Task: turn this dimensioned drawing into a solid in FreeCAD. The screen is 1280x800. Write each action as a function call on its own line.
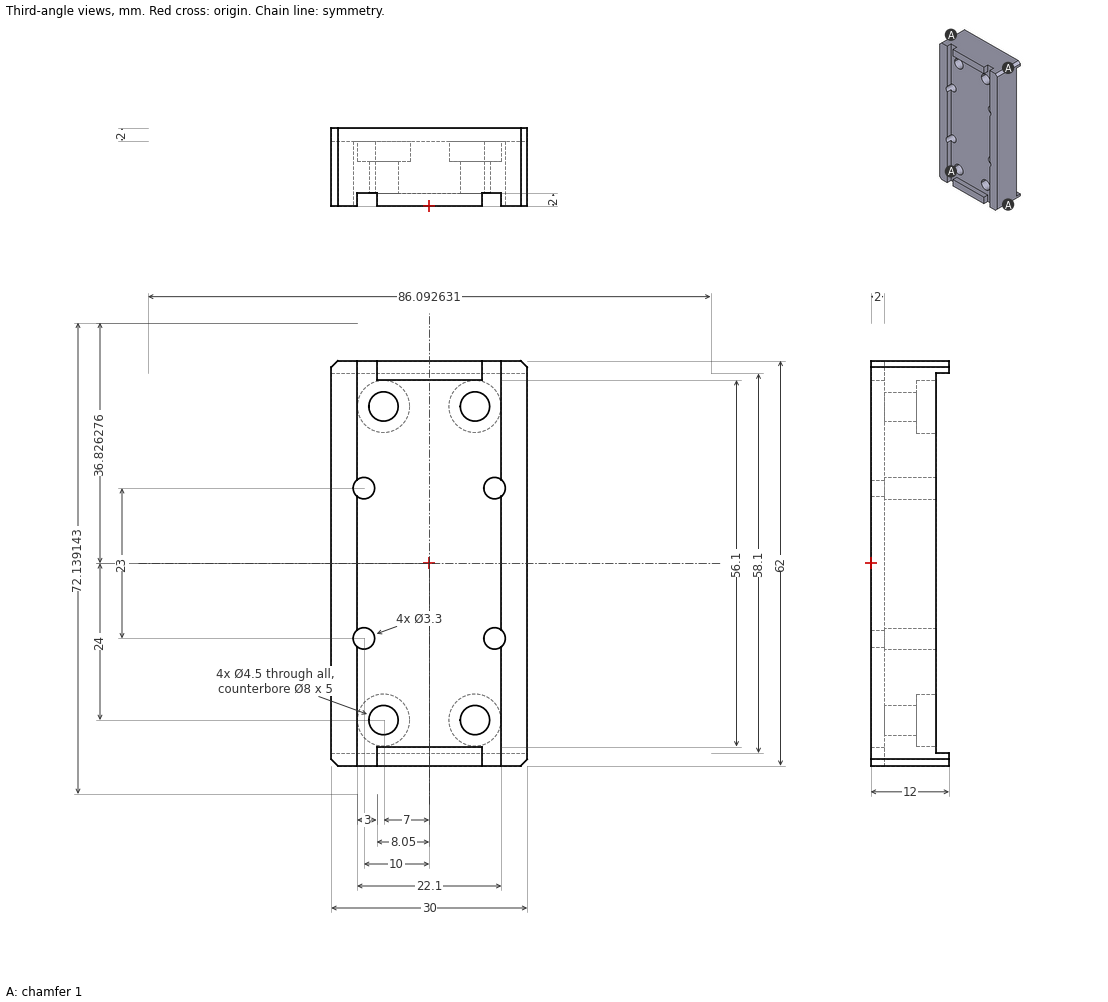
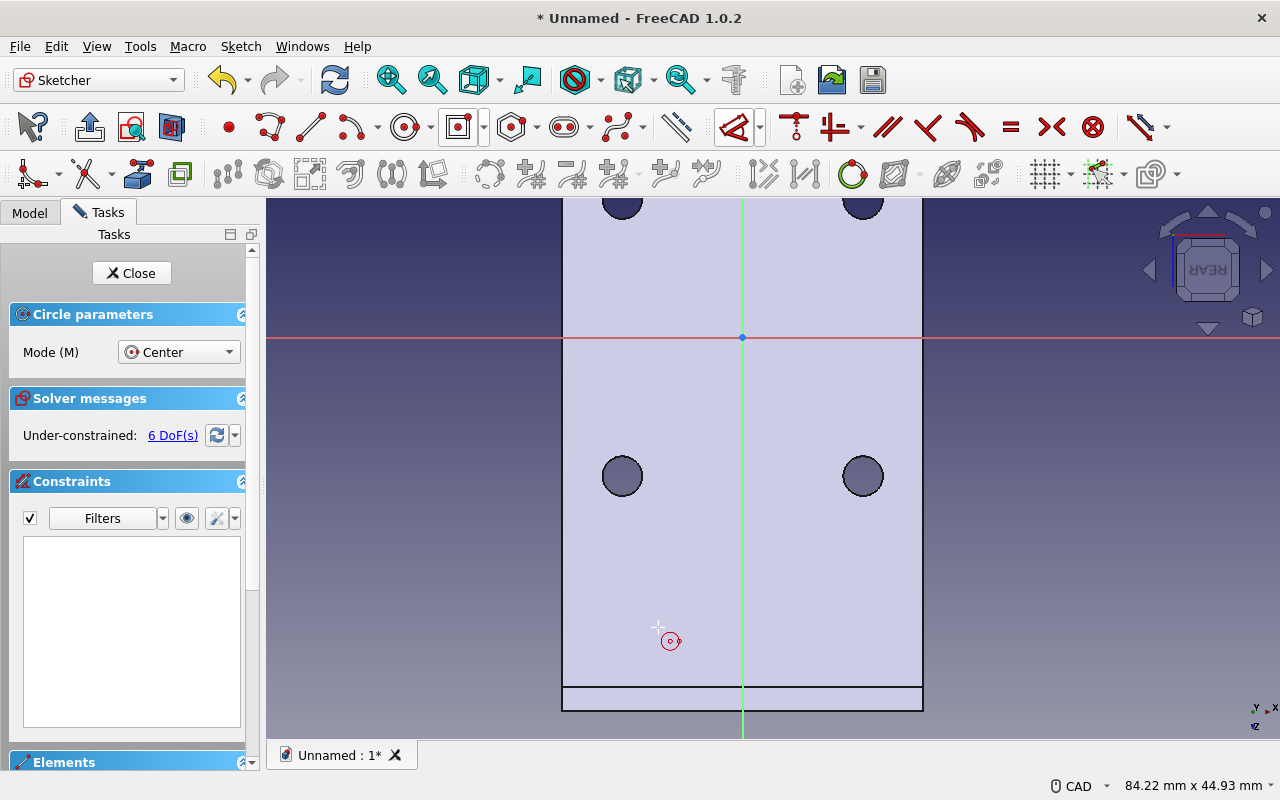
click(658, 627)
click(678, 607)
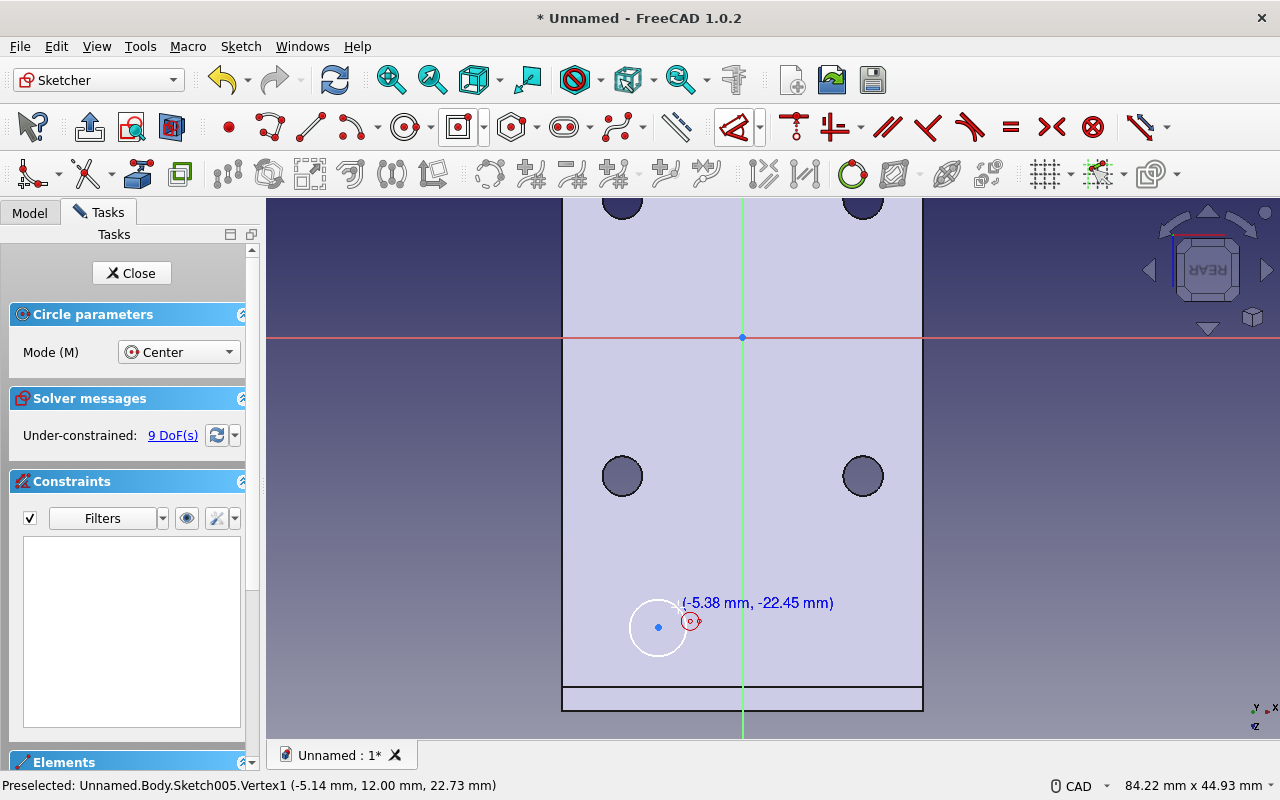
click(827, 627)
click(846, 607)
key(Escape)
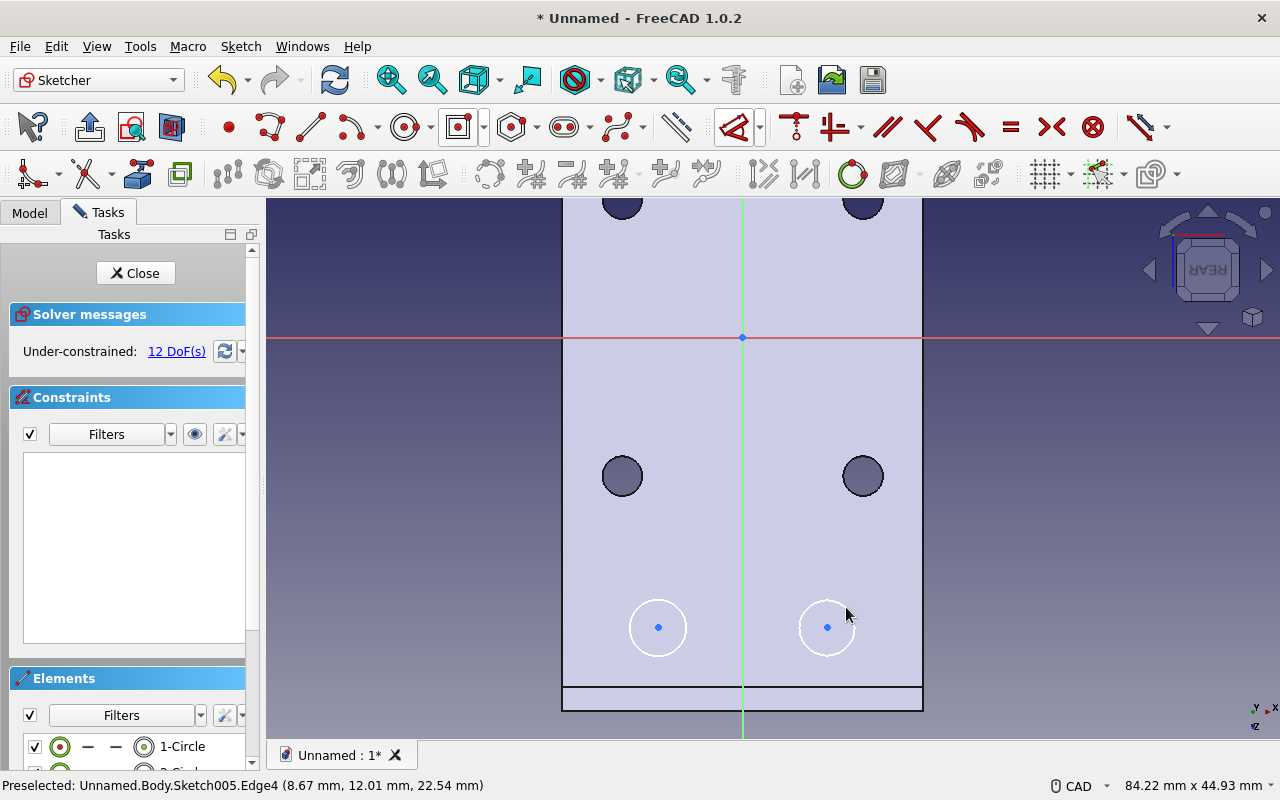
scroll(658, 628, down, 3)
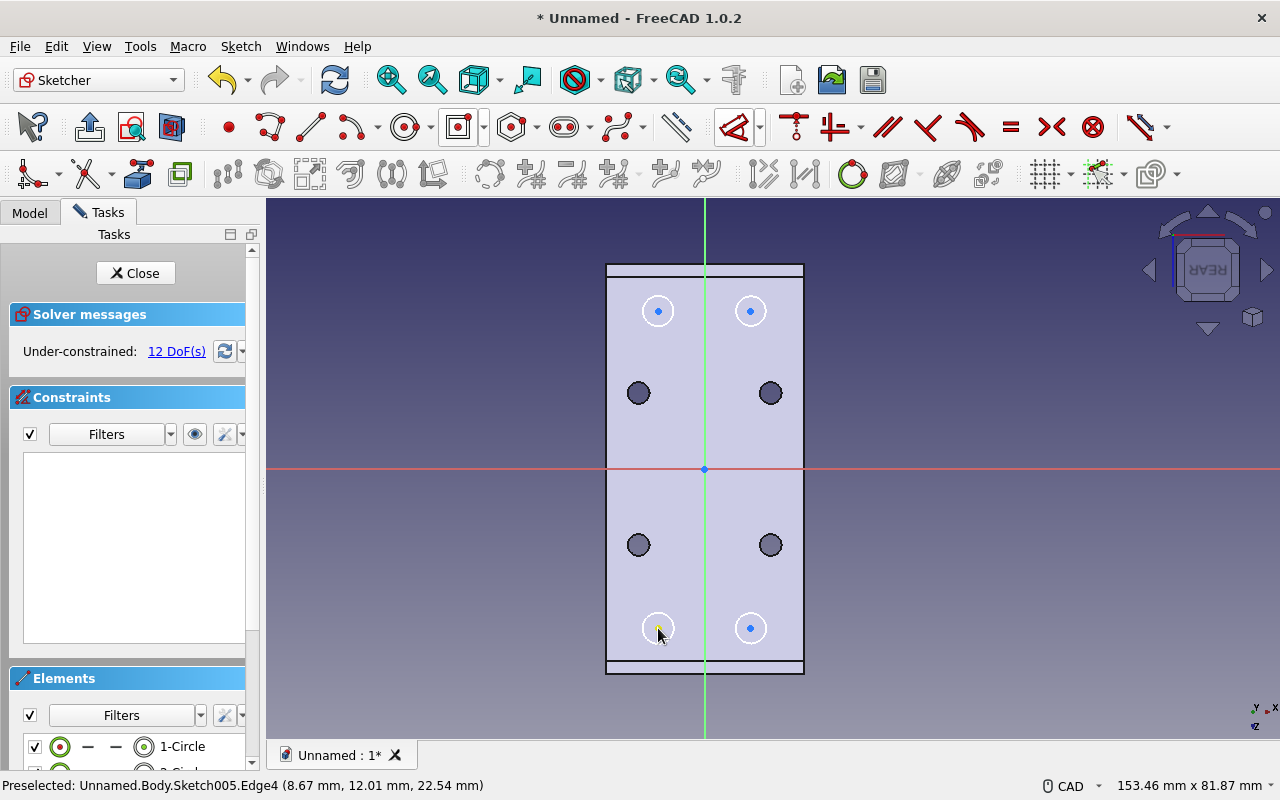
click(669, 300)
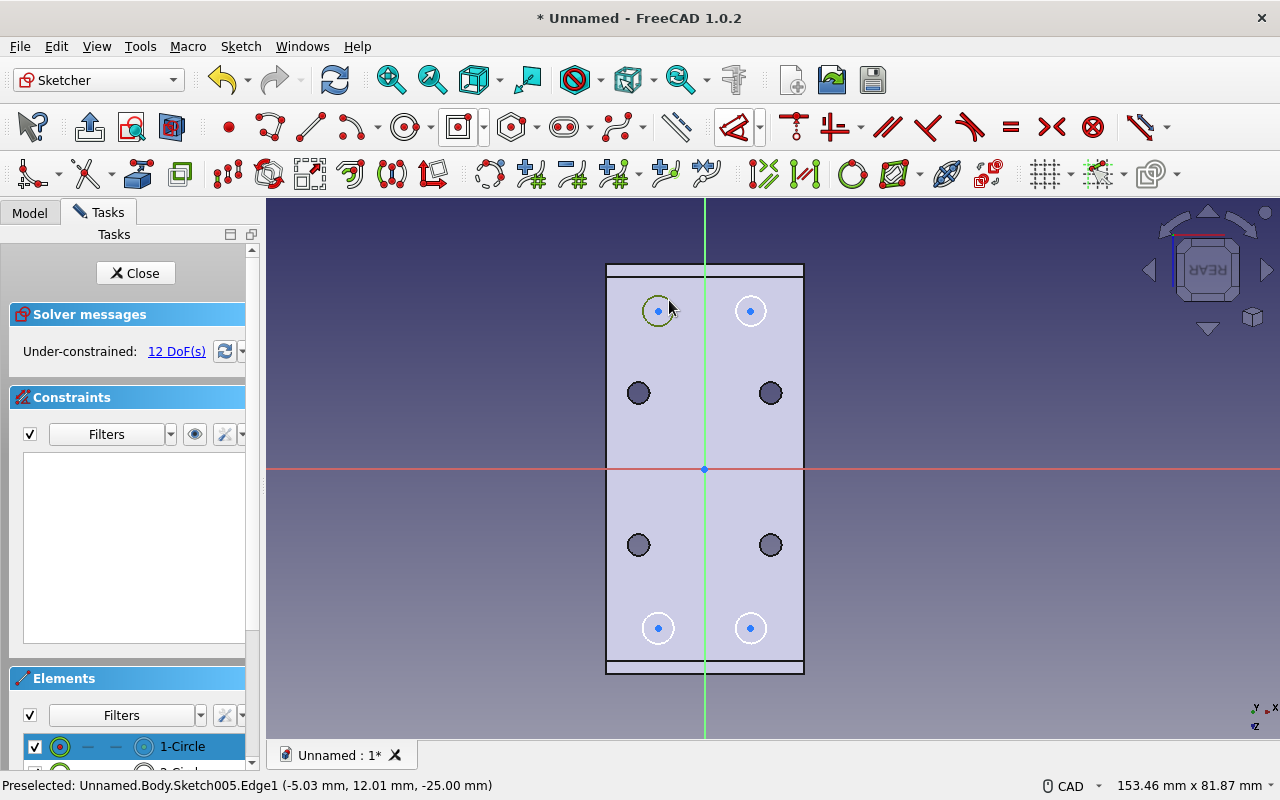
click(761, 301)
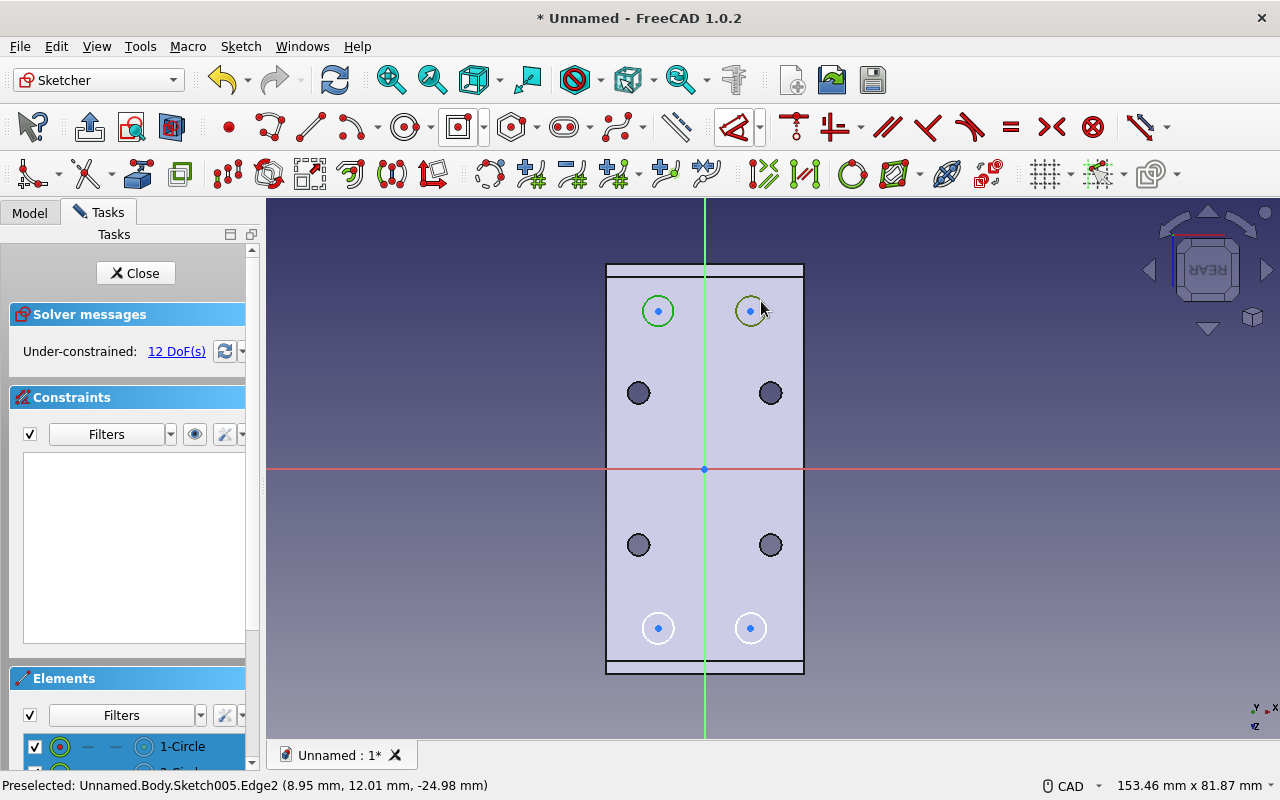
click(669, 617)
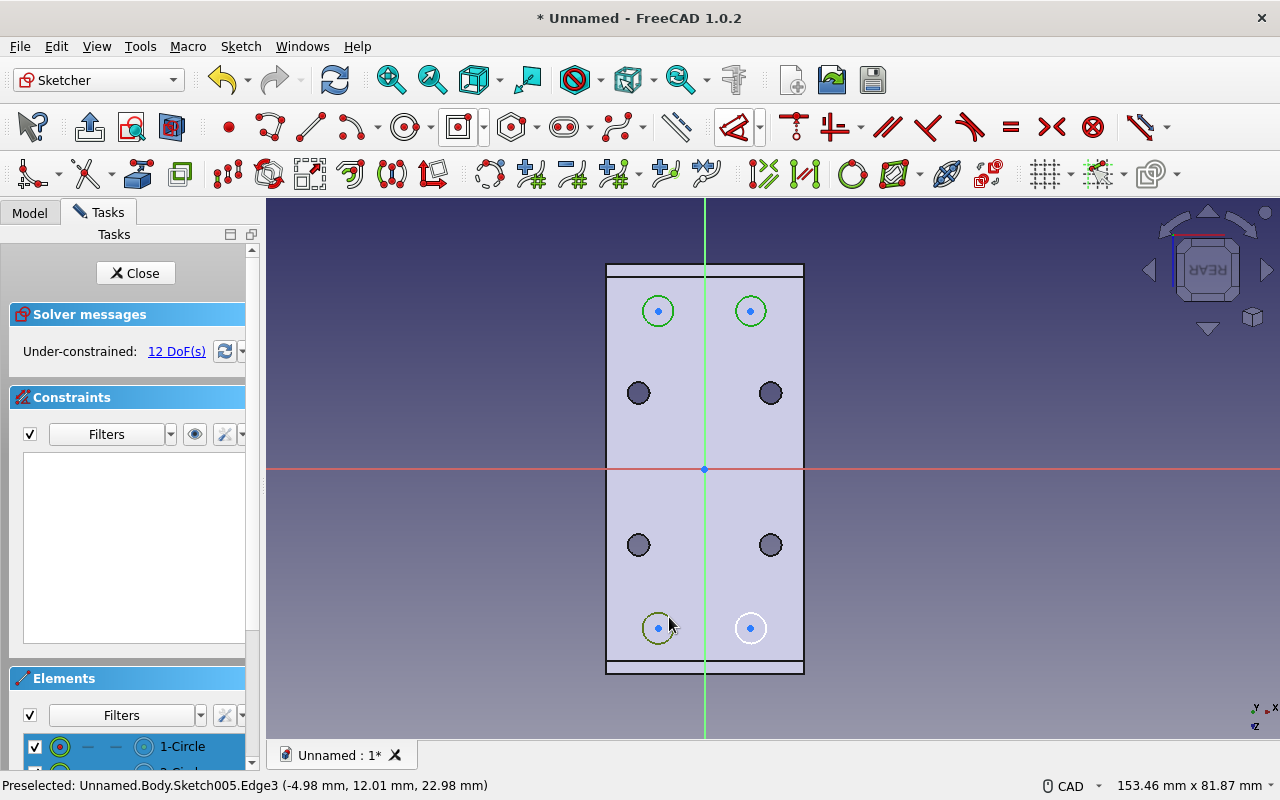
click(762, 618)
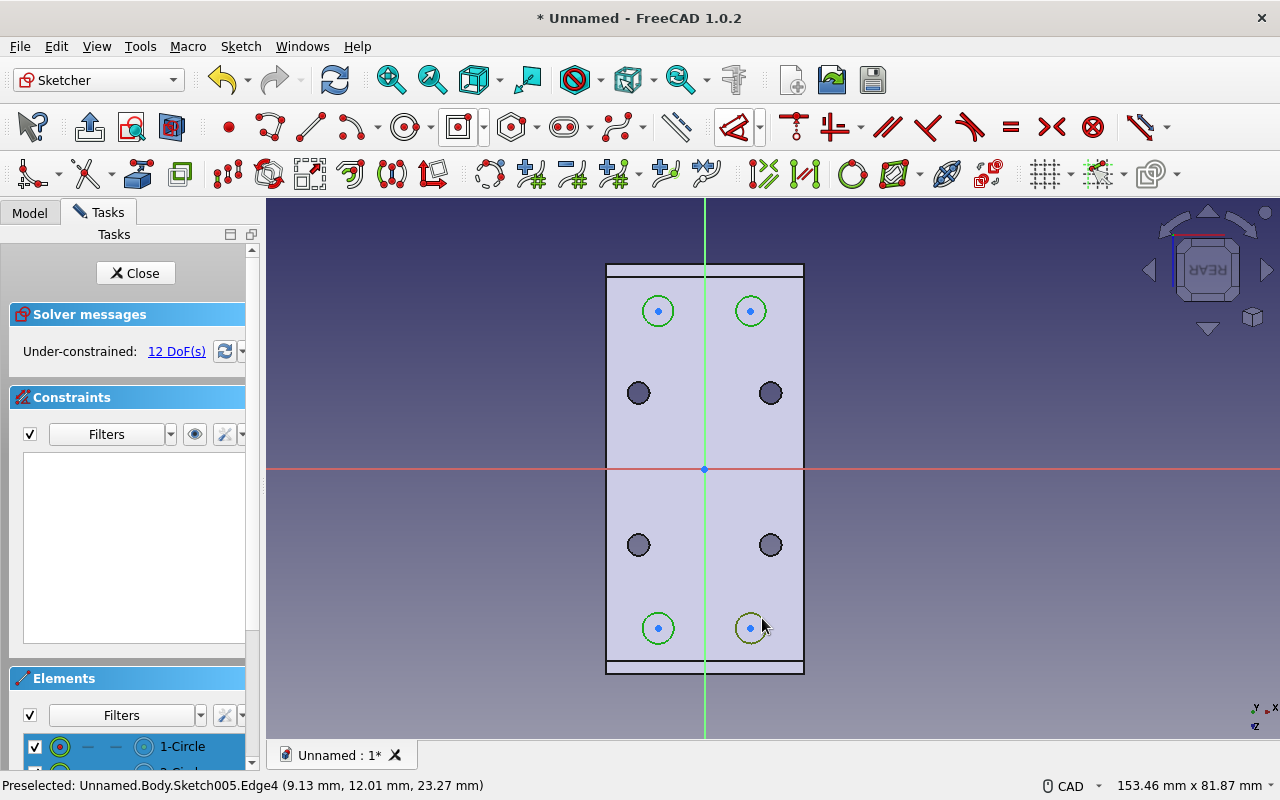
click(1011, 128)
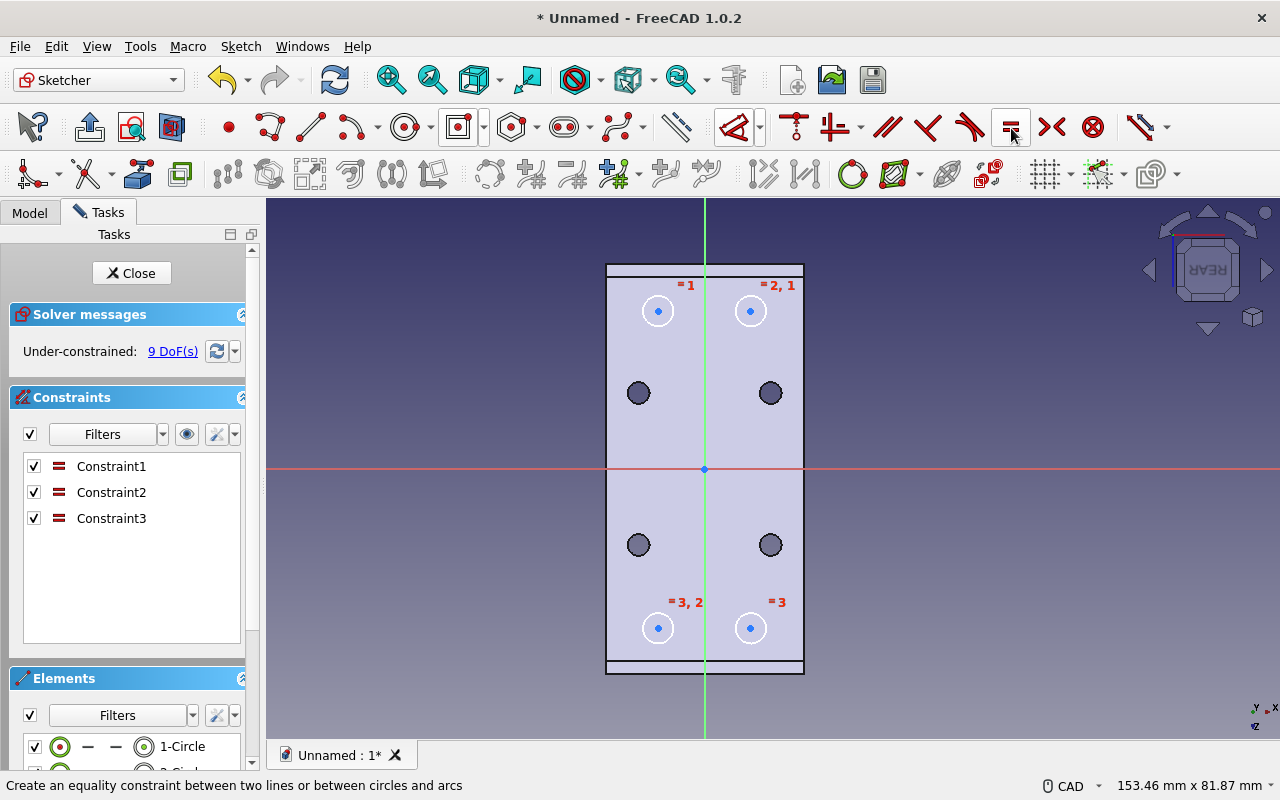
click(658, 311)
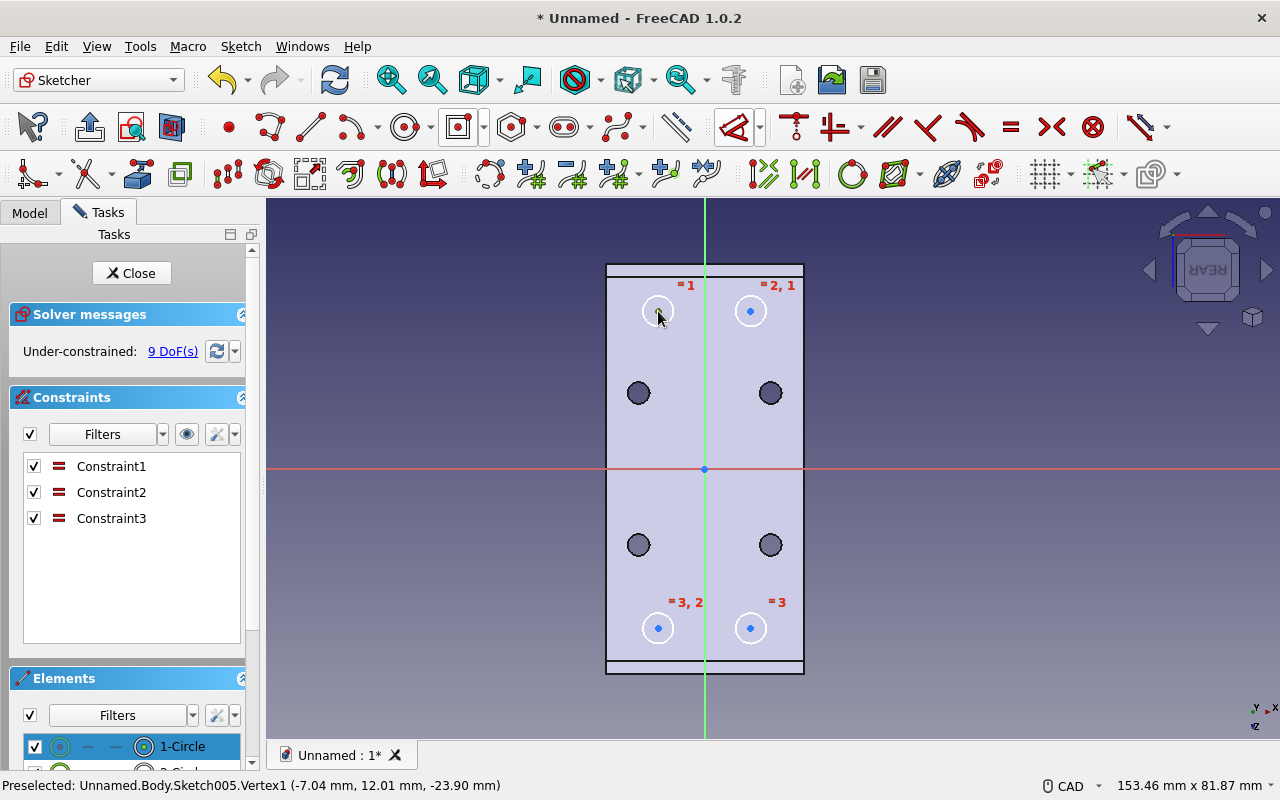
click(751, 311)